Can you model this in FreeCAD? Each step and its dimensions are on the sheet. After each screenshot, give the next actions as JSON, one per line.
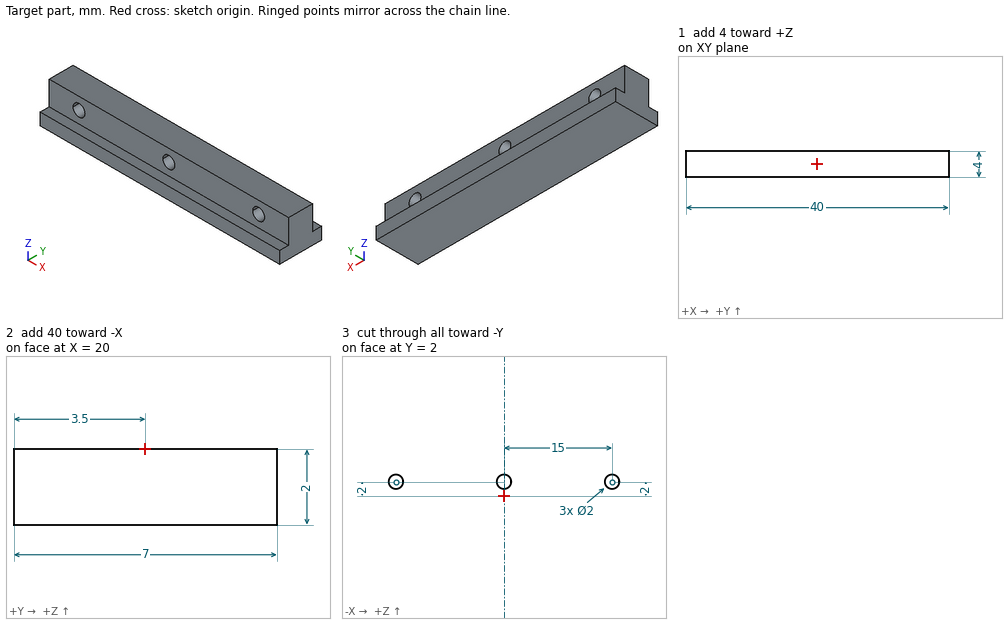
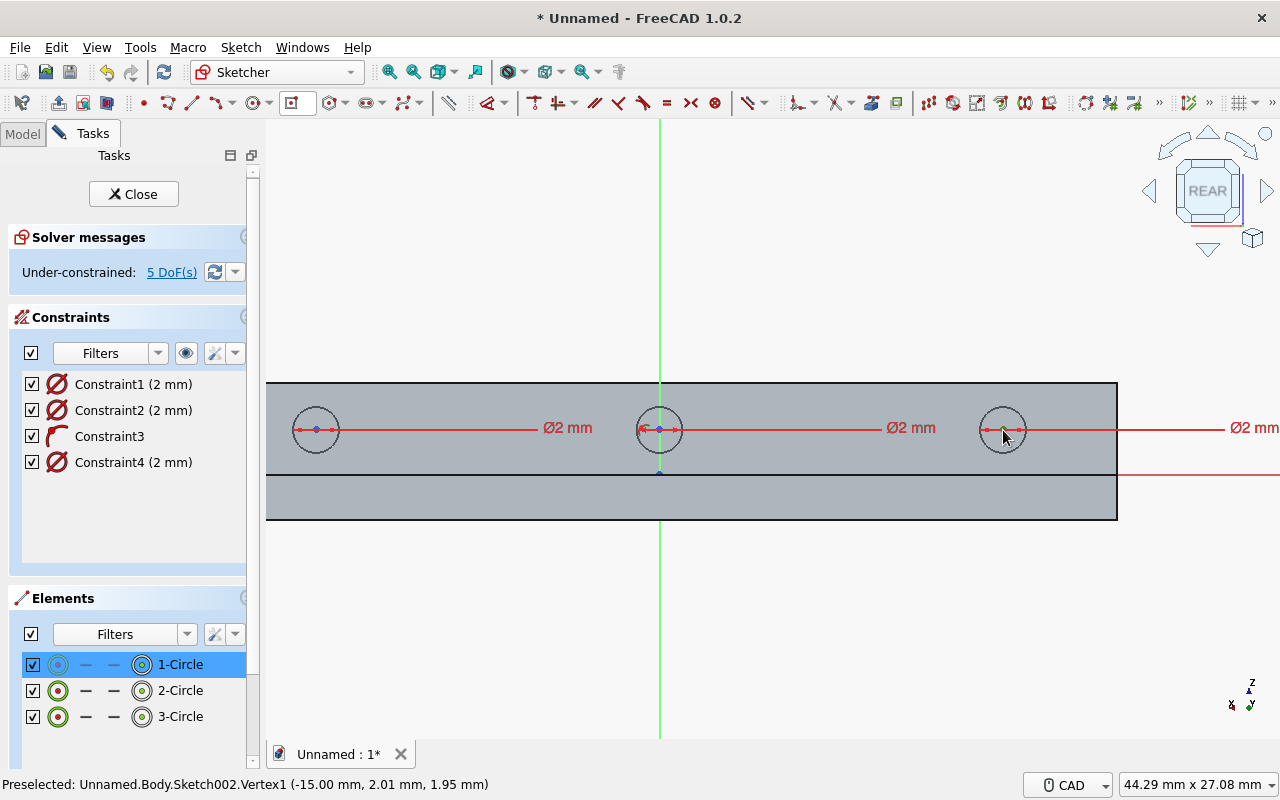
{"action": "left_click", "coordinate": [316, 430]}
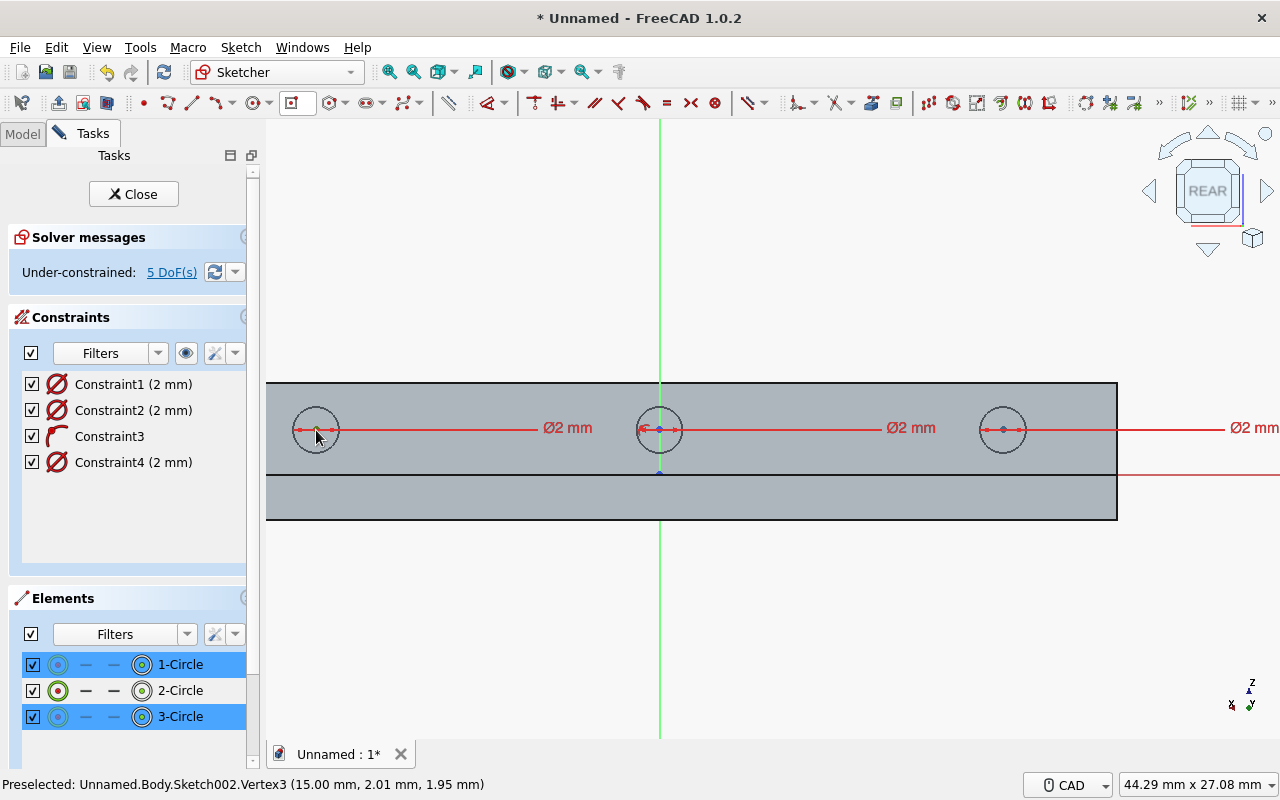
{"action": "left_click", "coordinate": [660, 671]}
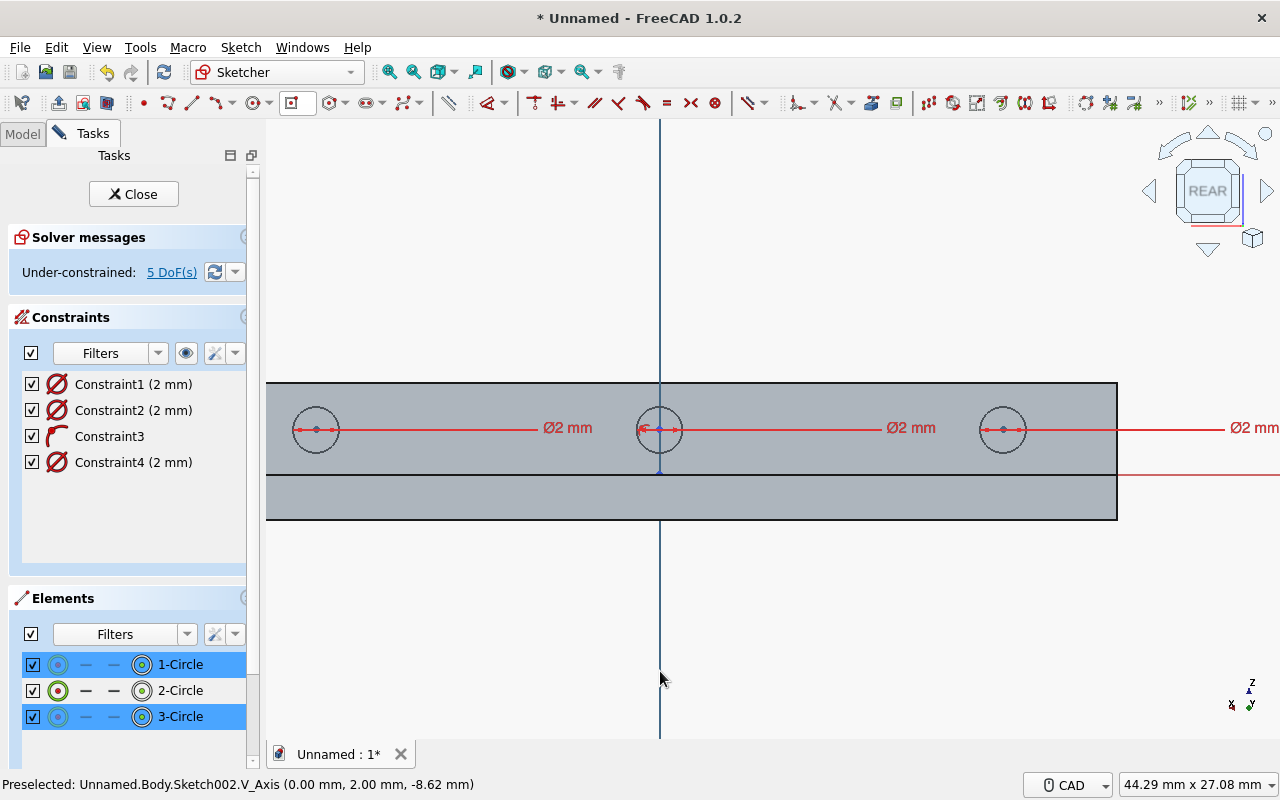
{"action": "key", "text": "s"}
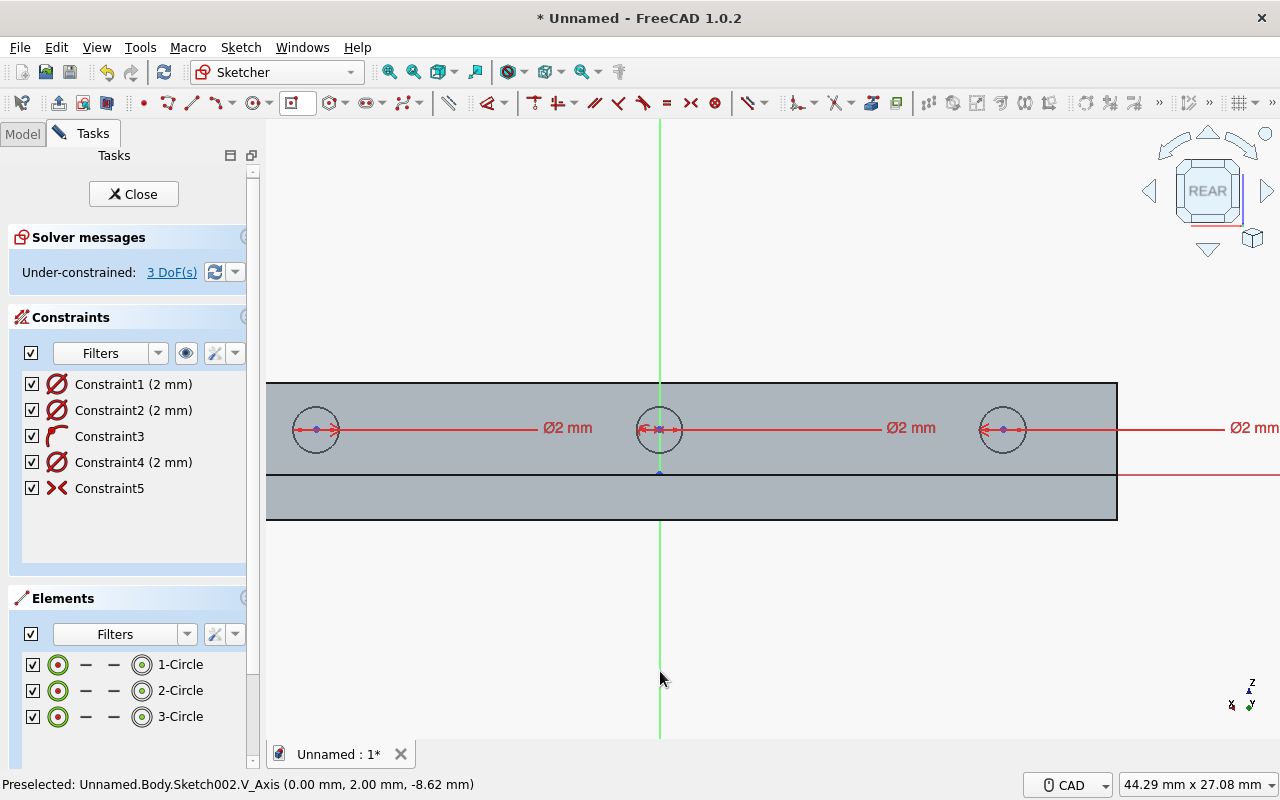
{"action": "key", "text": "d"}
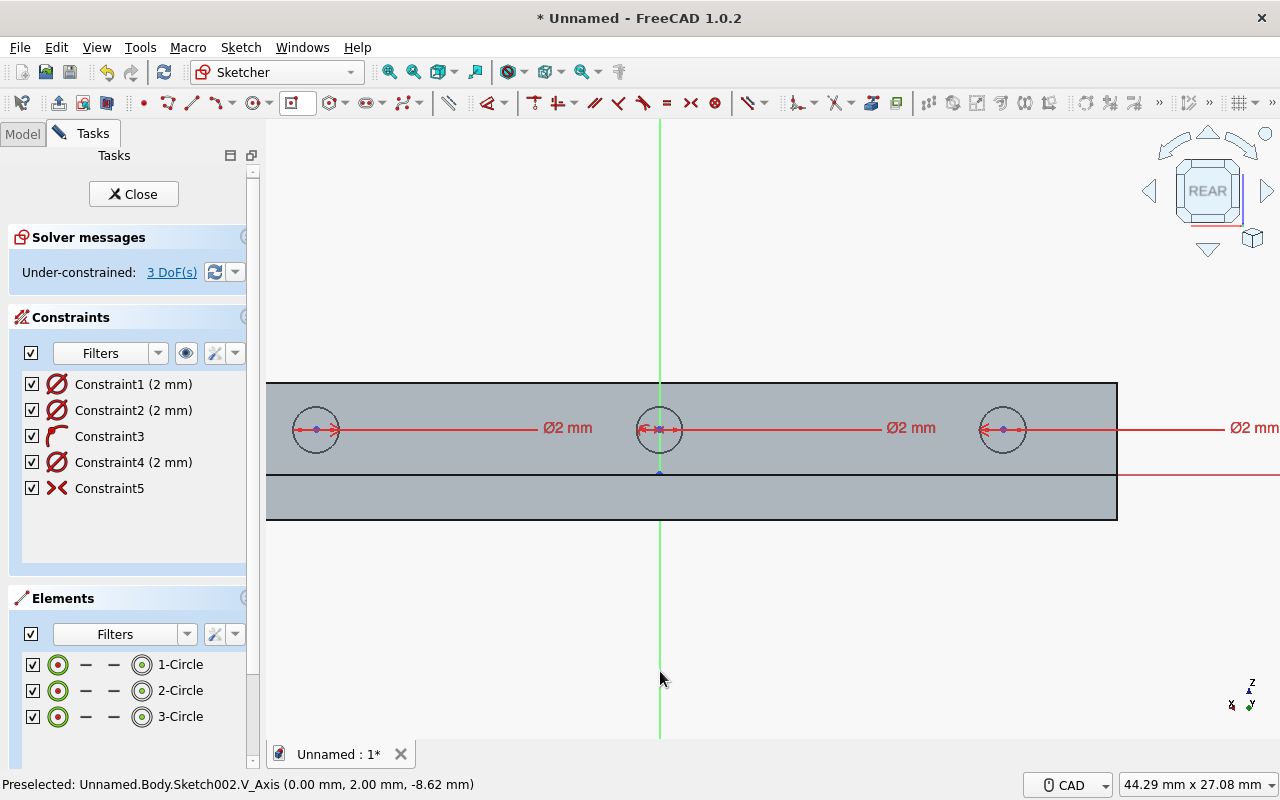
{"action": "left_click", "coordinate": [1003, 430]}
{"action": "left_click", "coordinate": [1037, 452]}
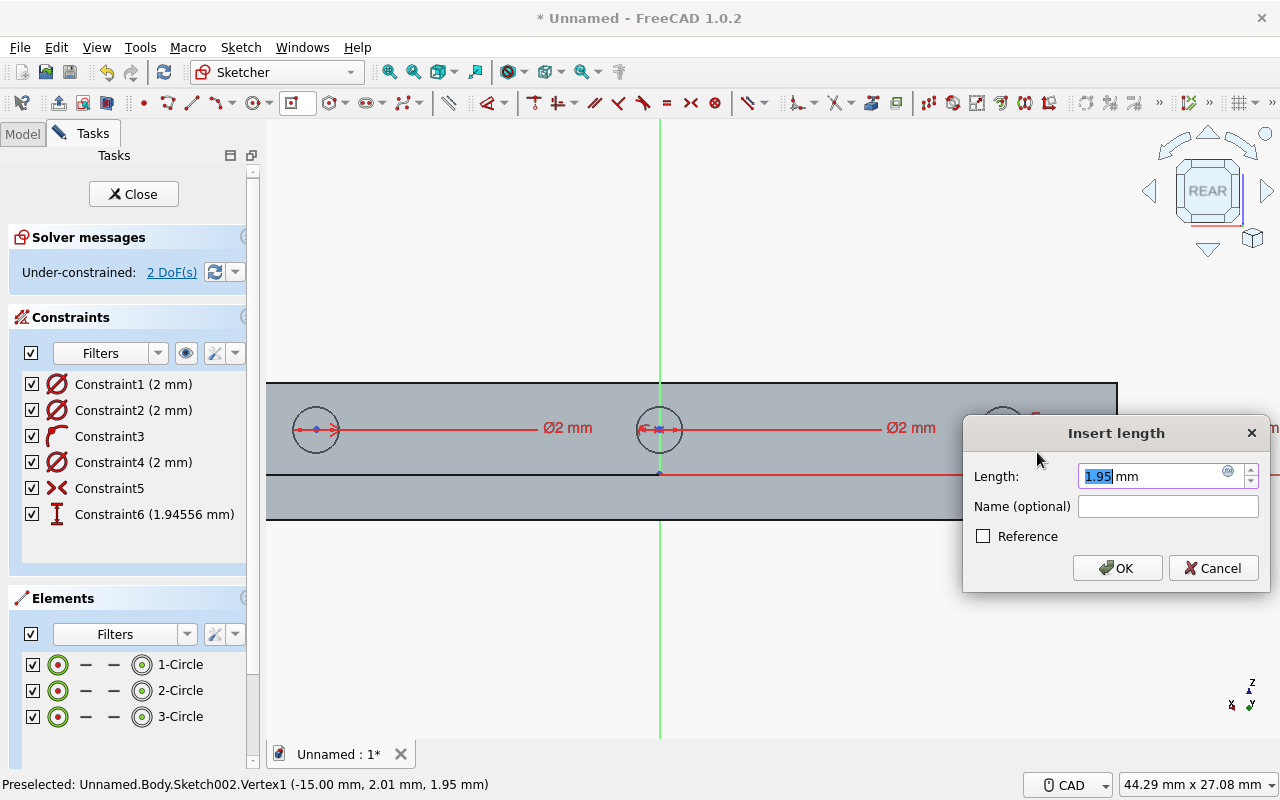
{"action": "type", "text": "2"}
{"action": "key", "text": "Return"}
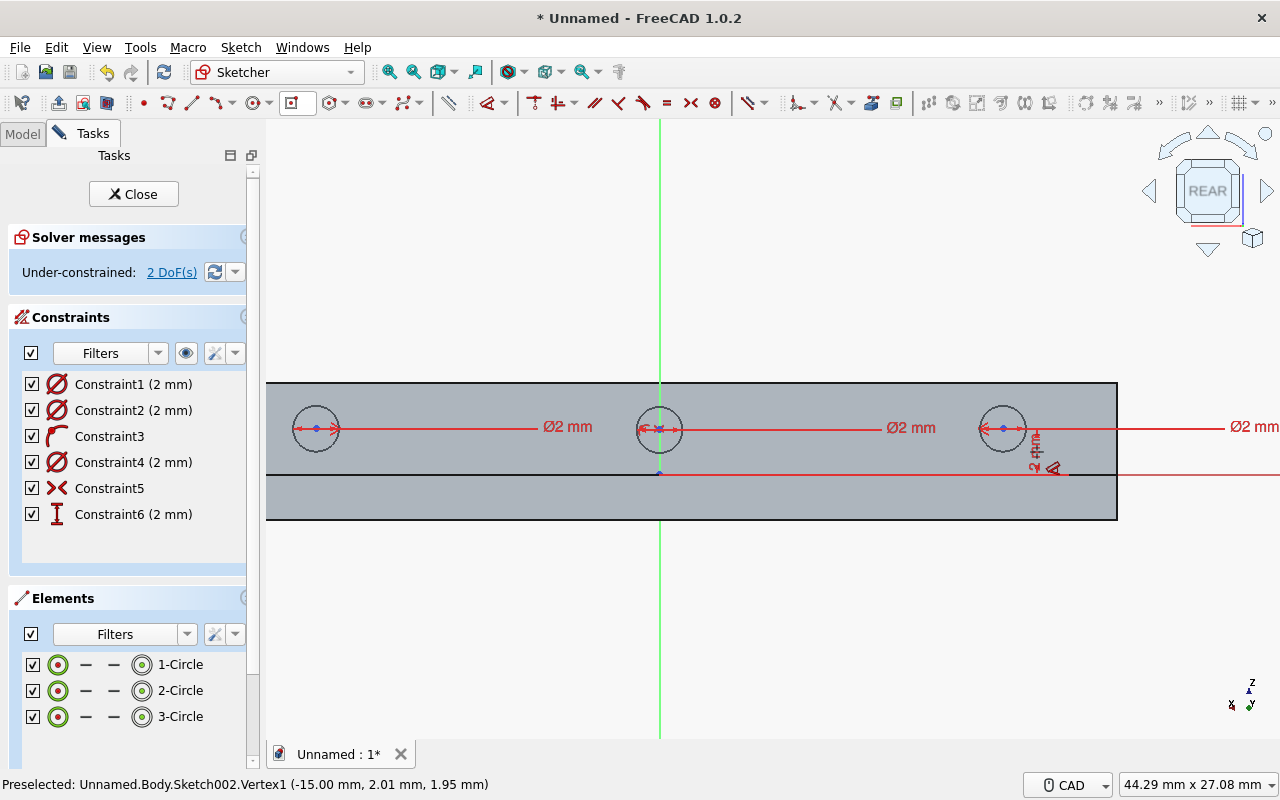
{"action": "left_click", "coordinate": [660, 430]}
{"action": "left_click", "coordinate": [694, 452]}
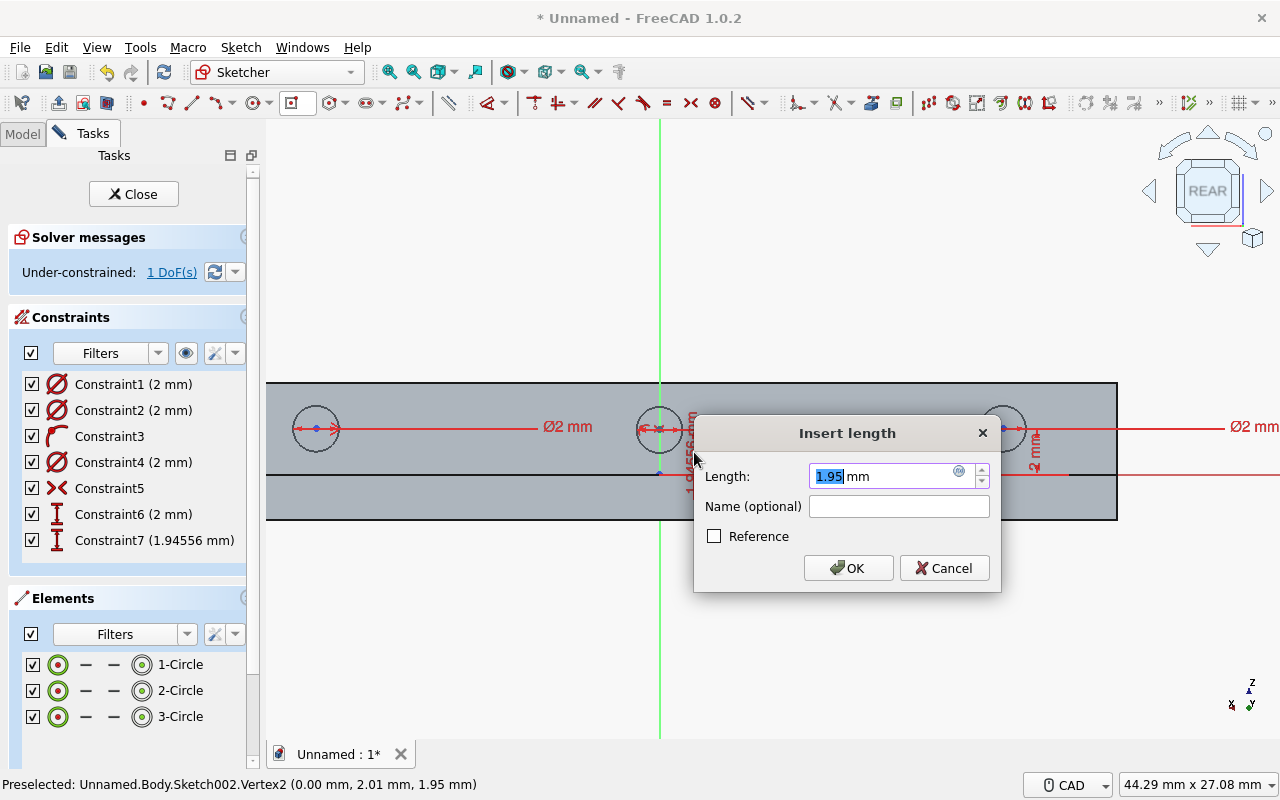
{"action": "type", "text": "2"}
{"action": "key", "text": "Return"}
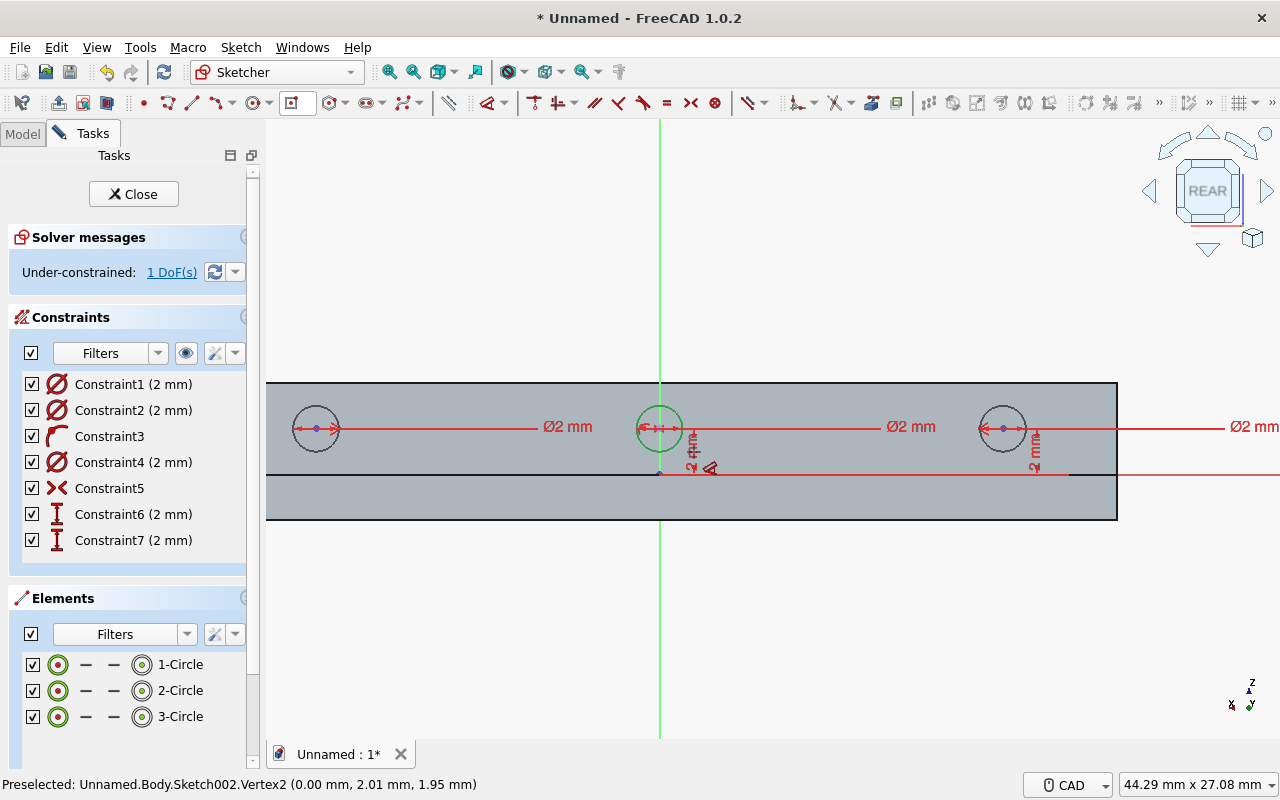
{"action": "left_click", "coordinate": [1003, 429]}
{"action": "left_click", "coordinate": [831, 509]}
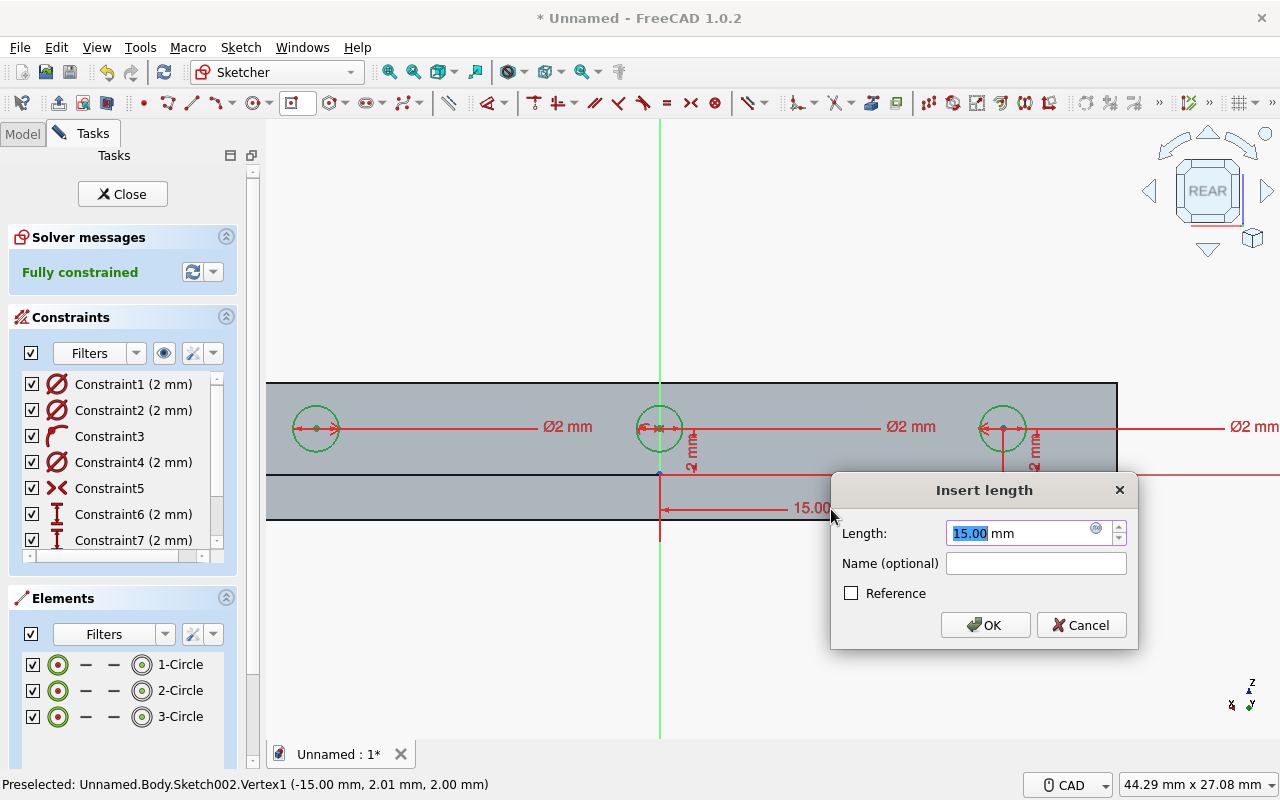
{"action": "type", "text": "15"}
{"action": "key", "text": "Return"}
{"action": "key", "text": "Escape"}